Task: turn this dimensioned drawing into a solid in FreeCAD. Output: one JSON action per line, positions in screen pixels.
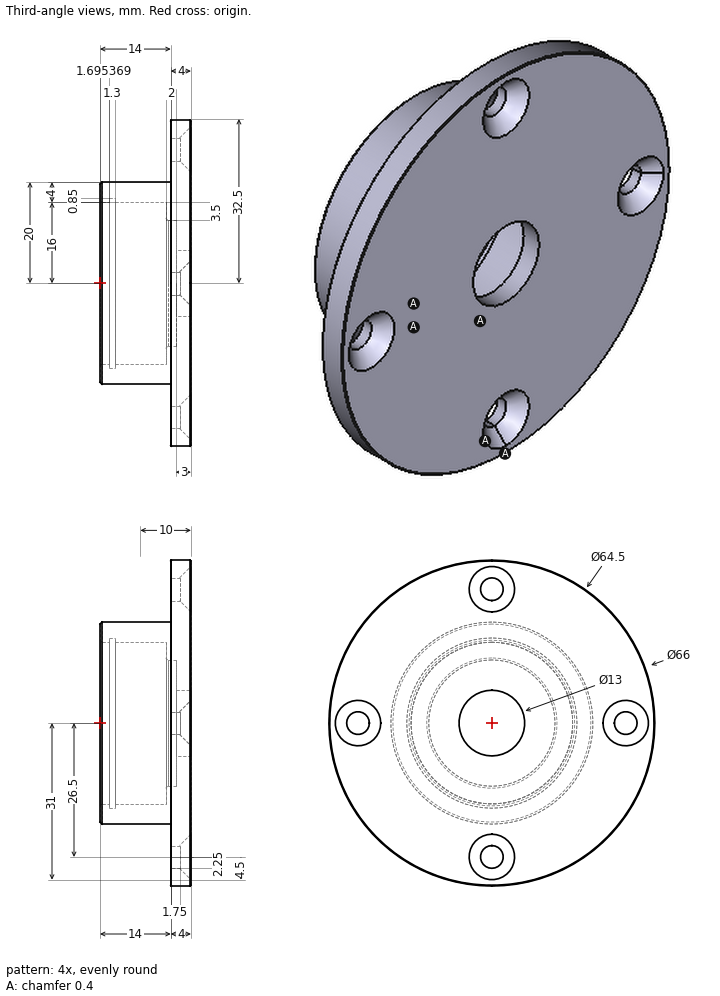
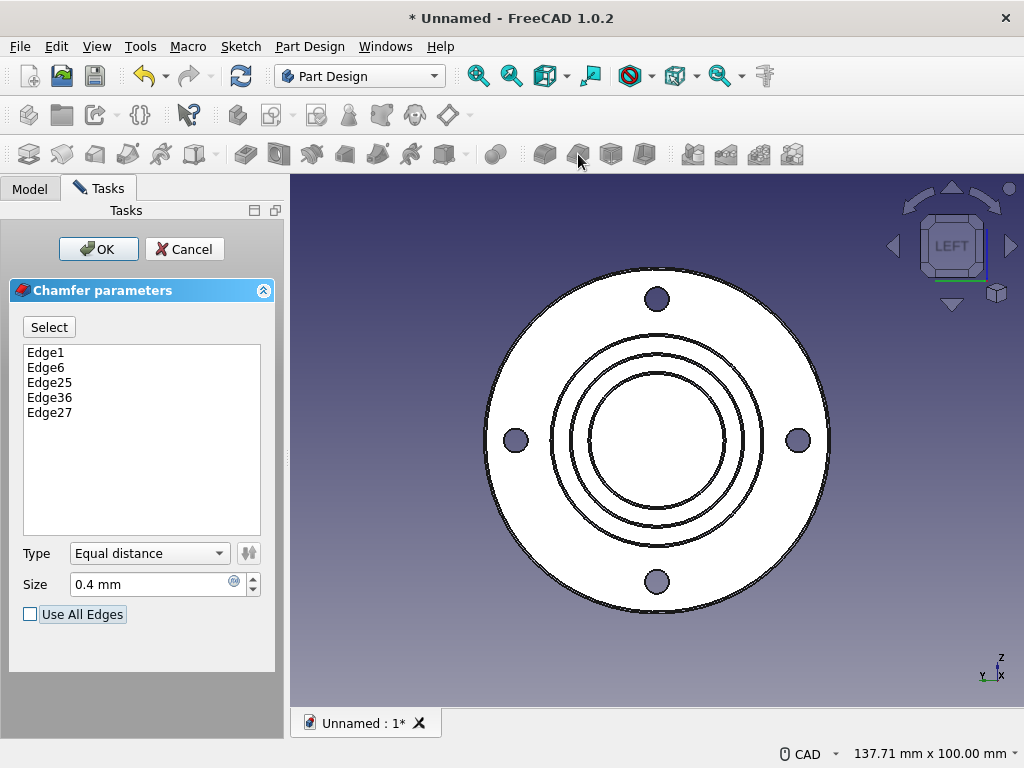
{"action": "left_click", "coordinate": [99, 249]}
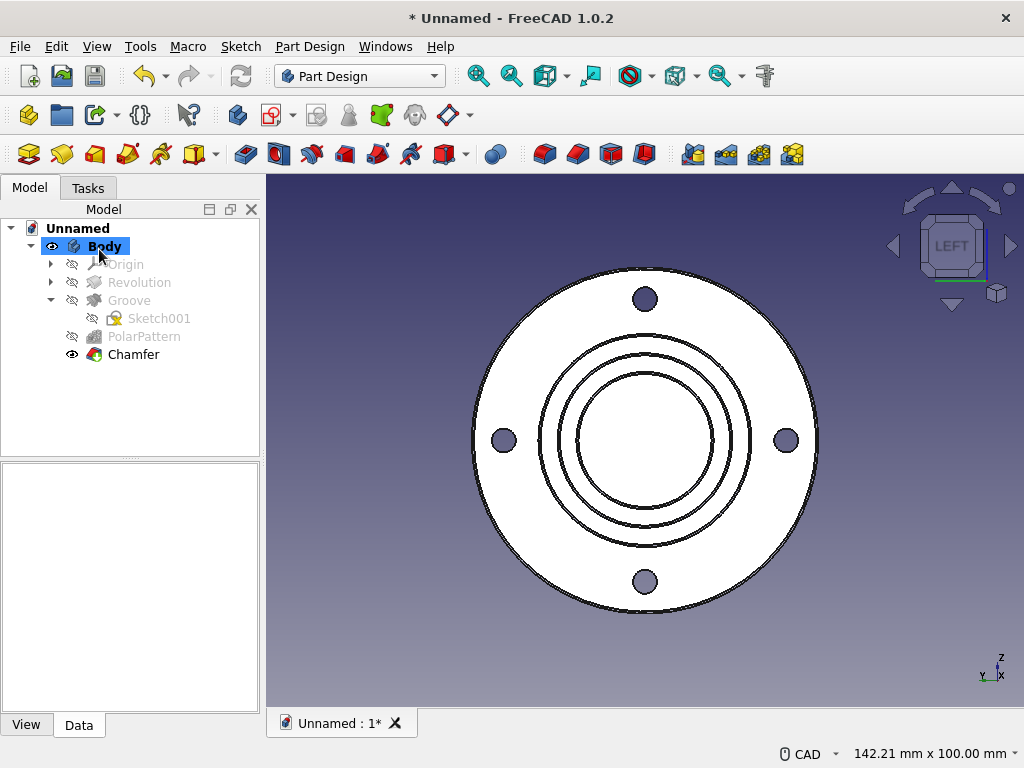
{"action": "left_click", "coordinate": [645, 439]}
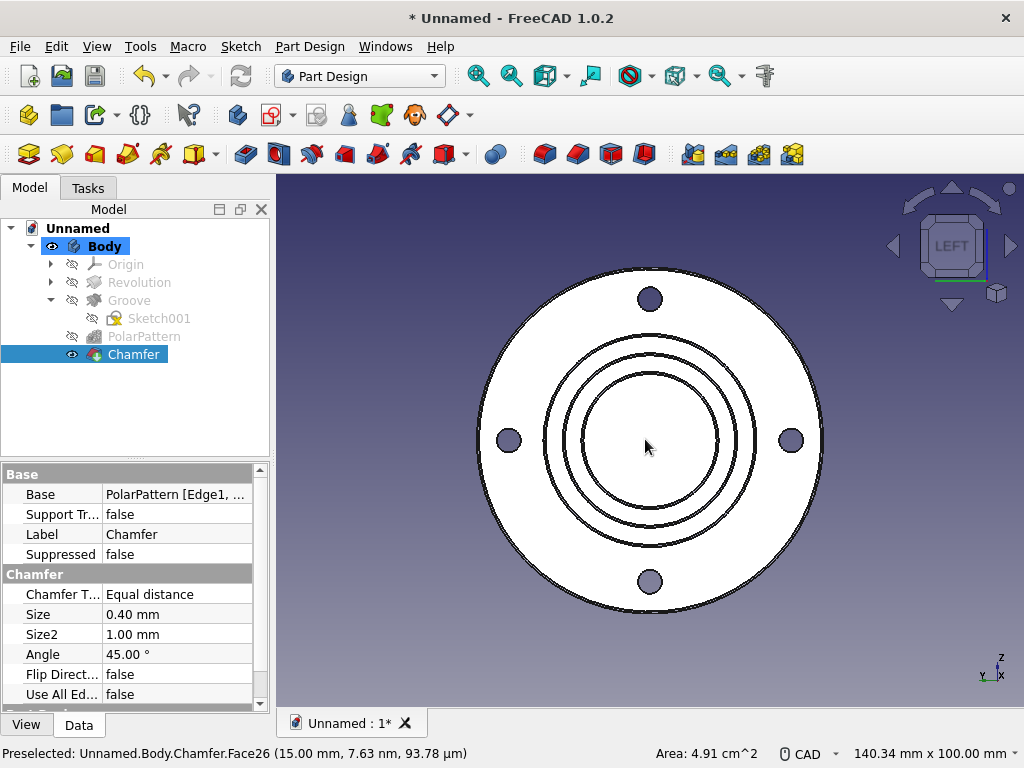
{"action": "left_click", "coordinate": [270, 116]}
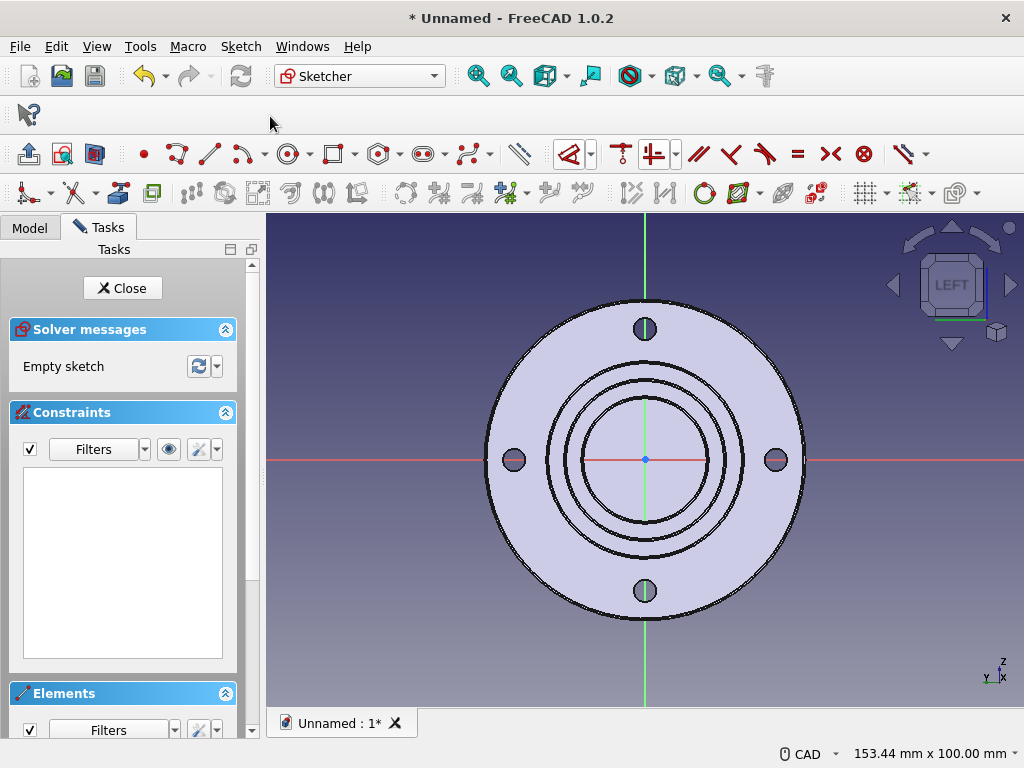
{"action": "left_click", "coordinate": [95, 154]}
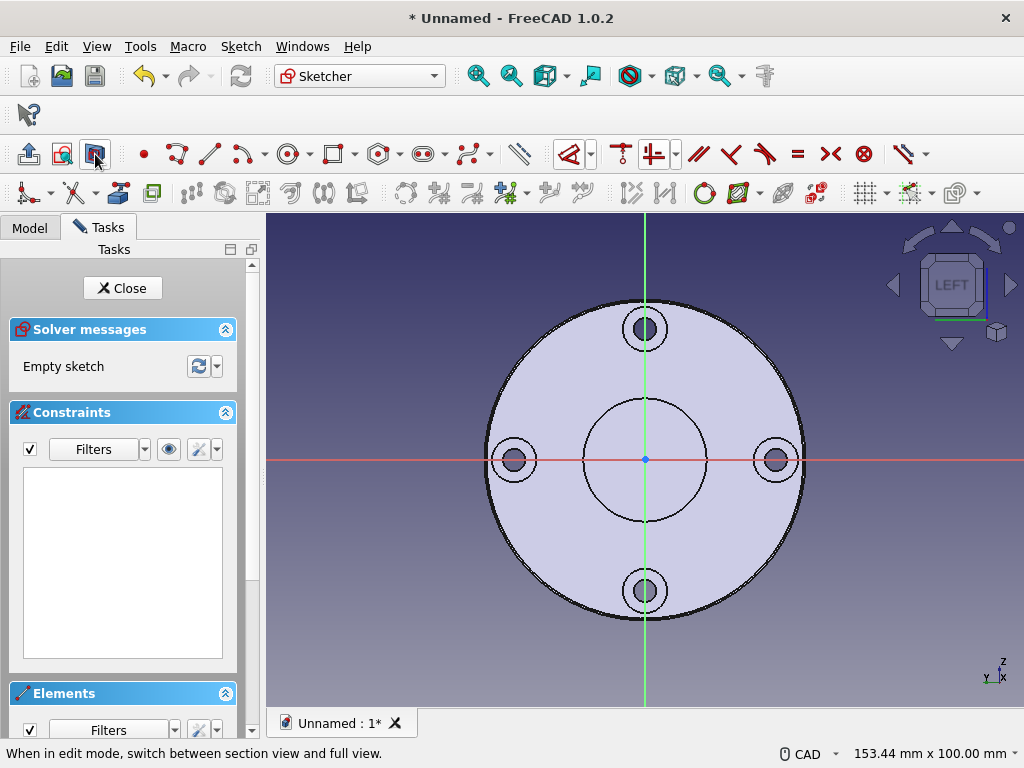
{"action": "scroll", "coordinate": [662, 460], "scroll_direction": "up", "scroll_amount": 8}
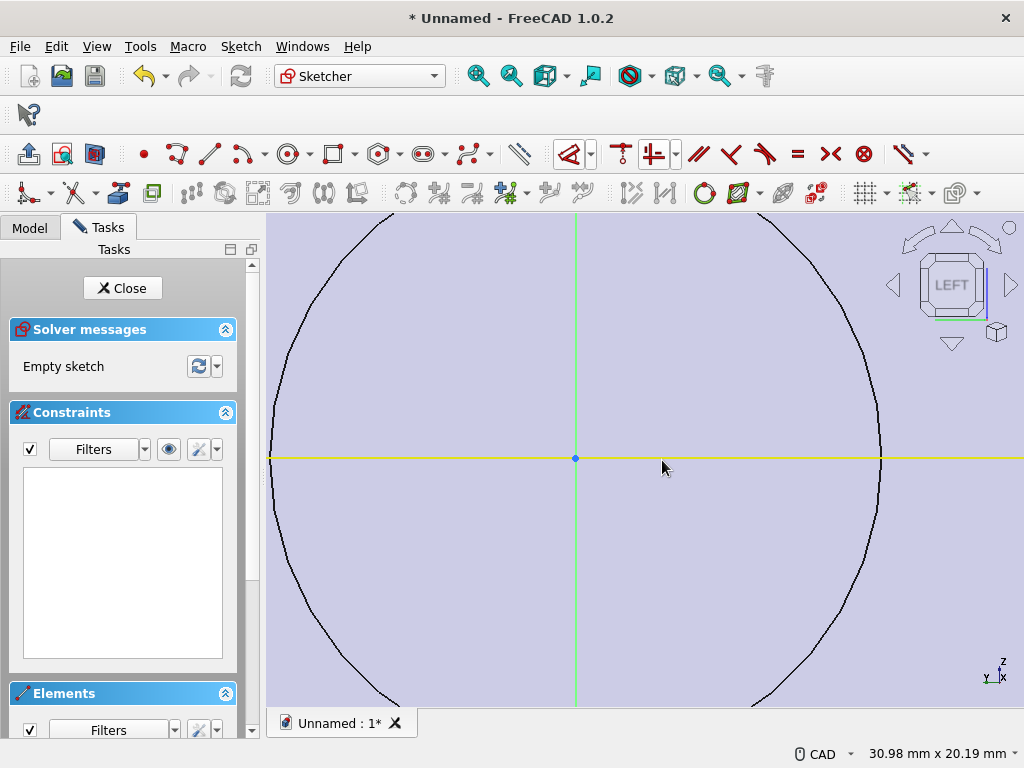
{"action": "left_click", "coordinate": [288, 154]}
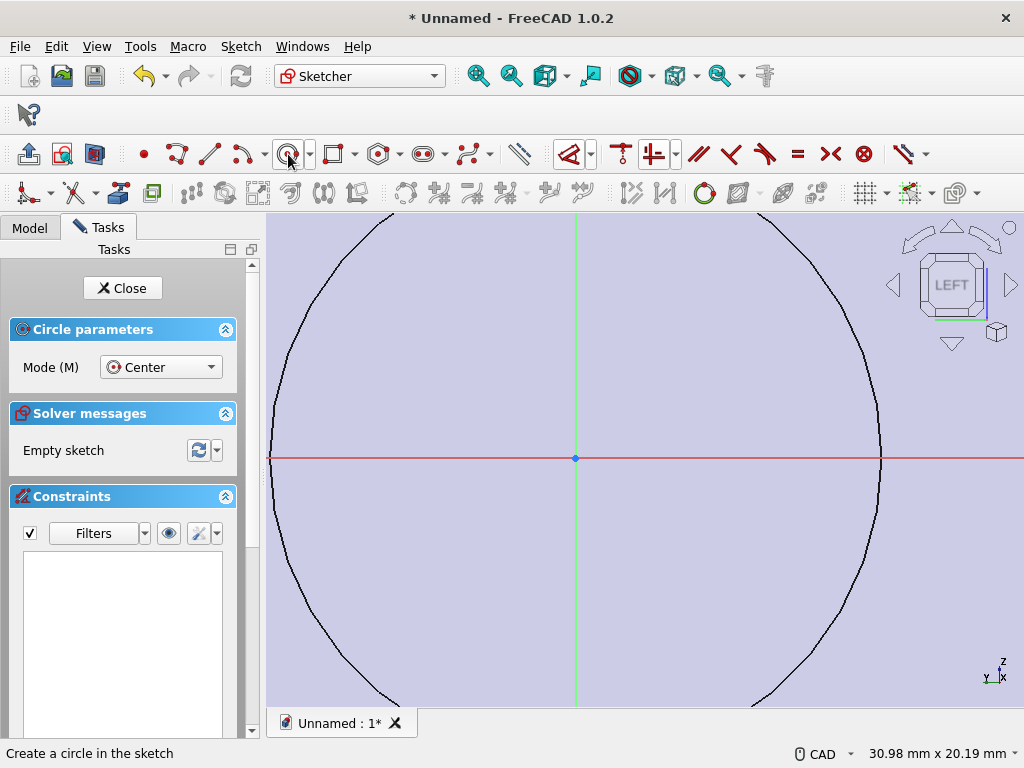
{"action": "left_click", "coordinate": [576, 458]}
{"action": "mouse_move", "coordinate": [688, 346]}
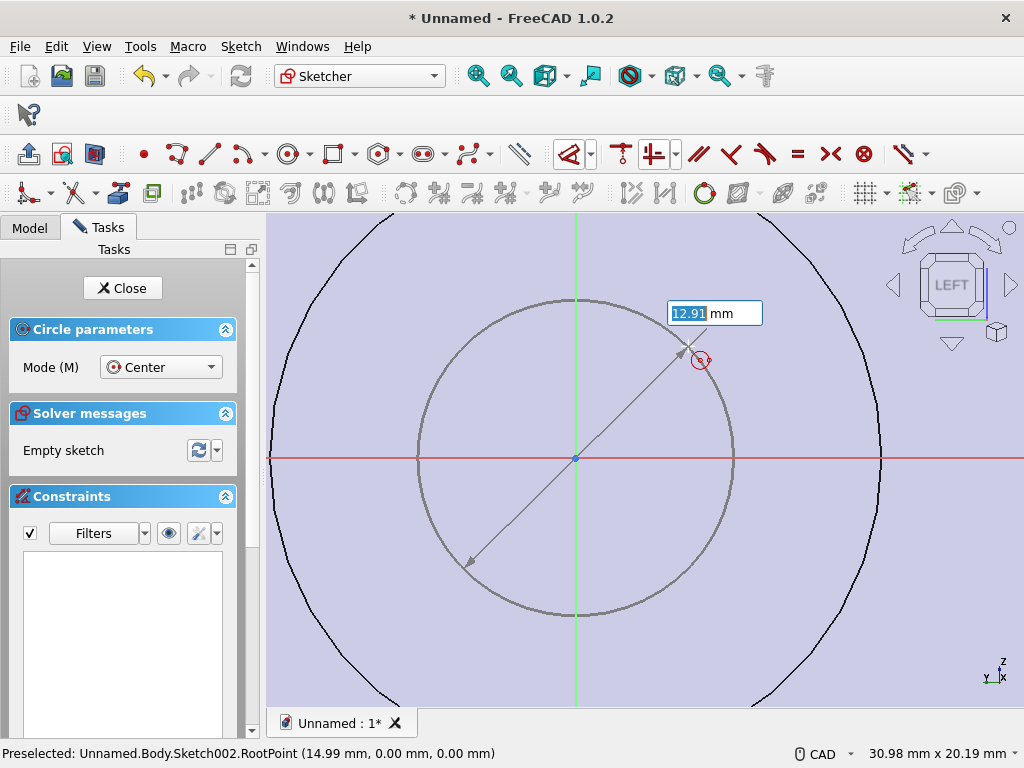
{"action": "type", "text": "13"}
{"action": "key", "text": "Return"}
{"action": "key", "text": "Escape"}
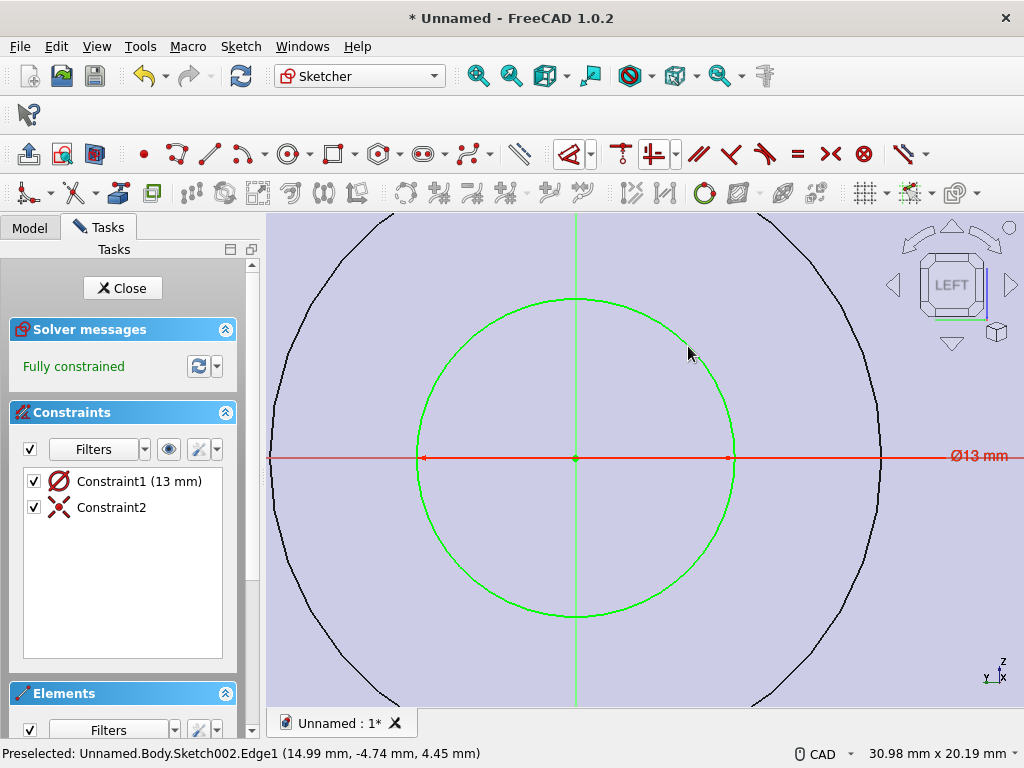
{"action": "left_click", "coordinate": [123, 288]}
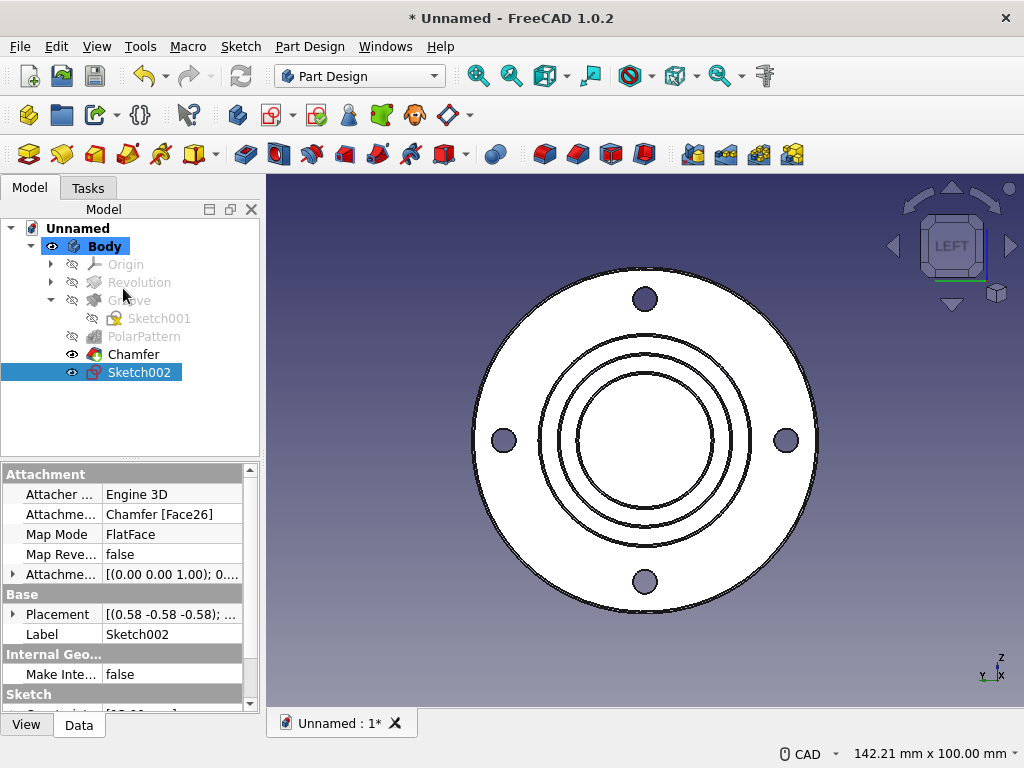
{"action": "left_click", "coordinate": [246, 154]}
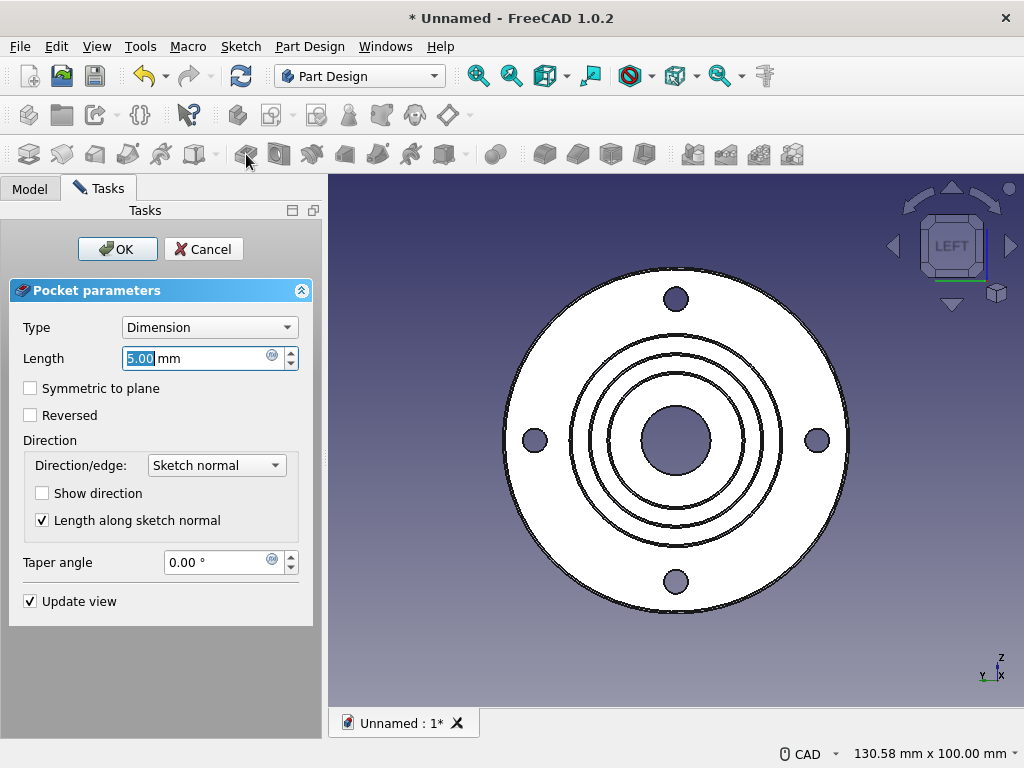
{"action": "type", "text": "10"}
{"action": "key", "text": "Tab"}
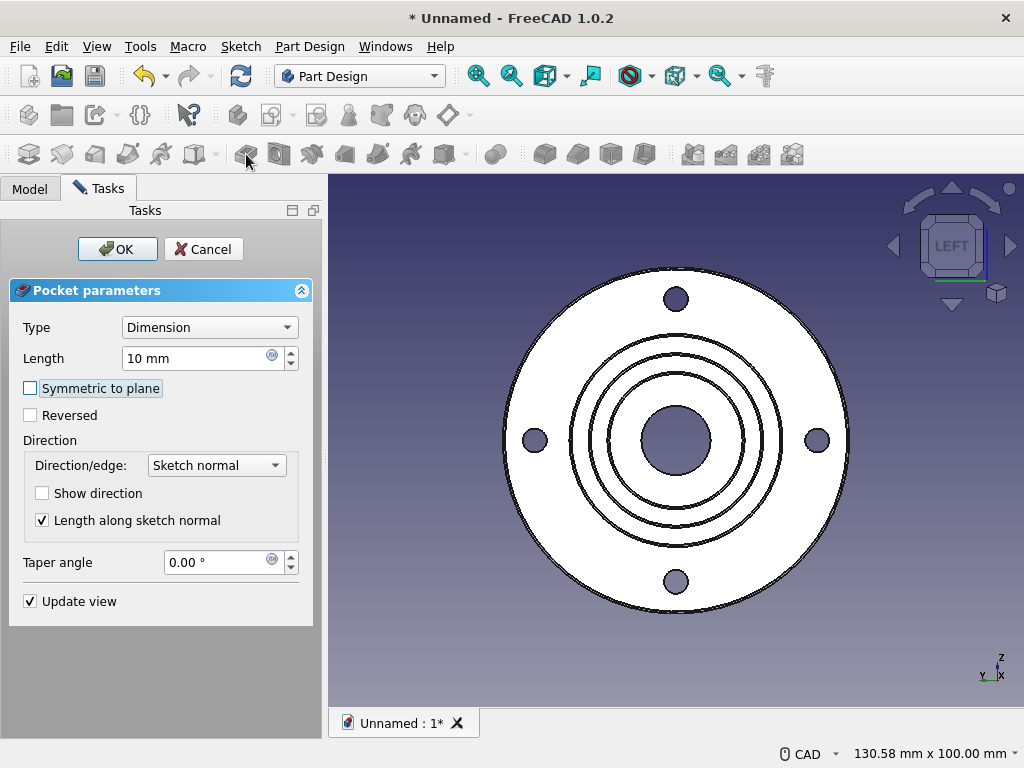
{"action": "left_click", "coordinate": [118, 249]}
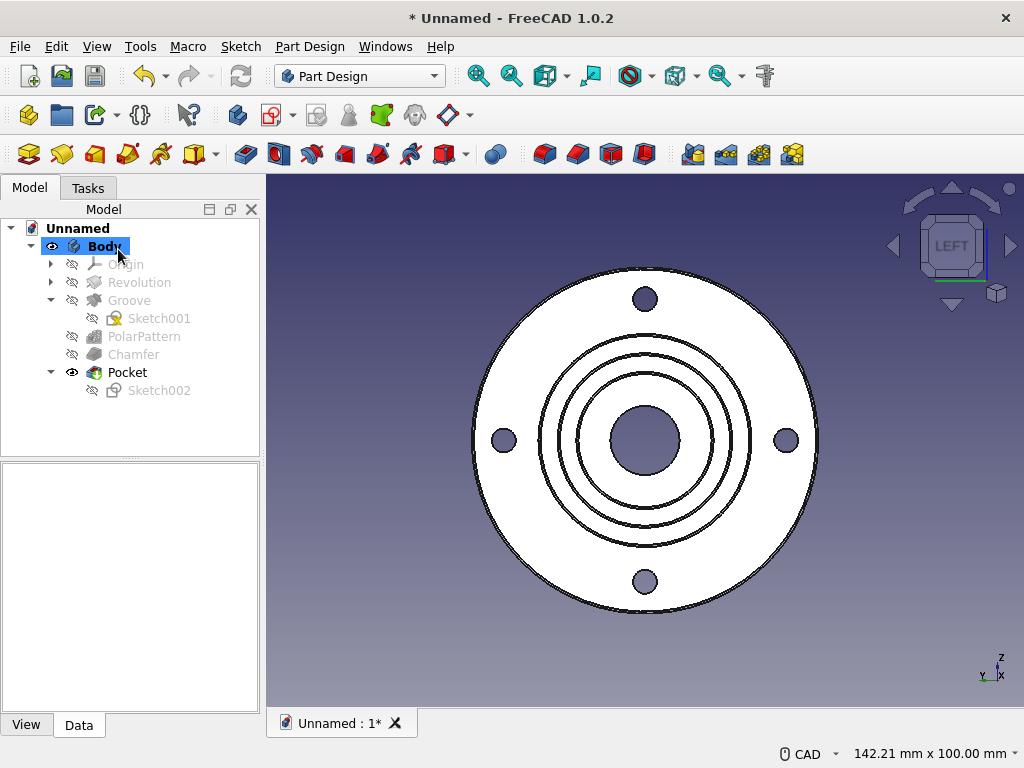
{"action": "key", "text": "0"}